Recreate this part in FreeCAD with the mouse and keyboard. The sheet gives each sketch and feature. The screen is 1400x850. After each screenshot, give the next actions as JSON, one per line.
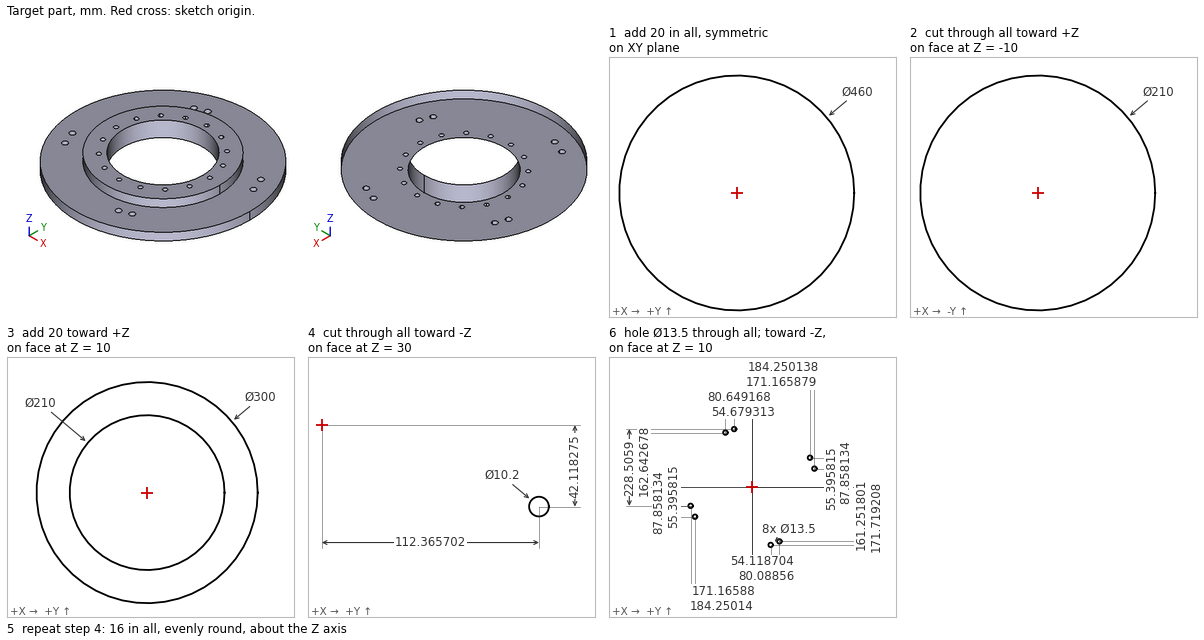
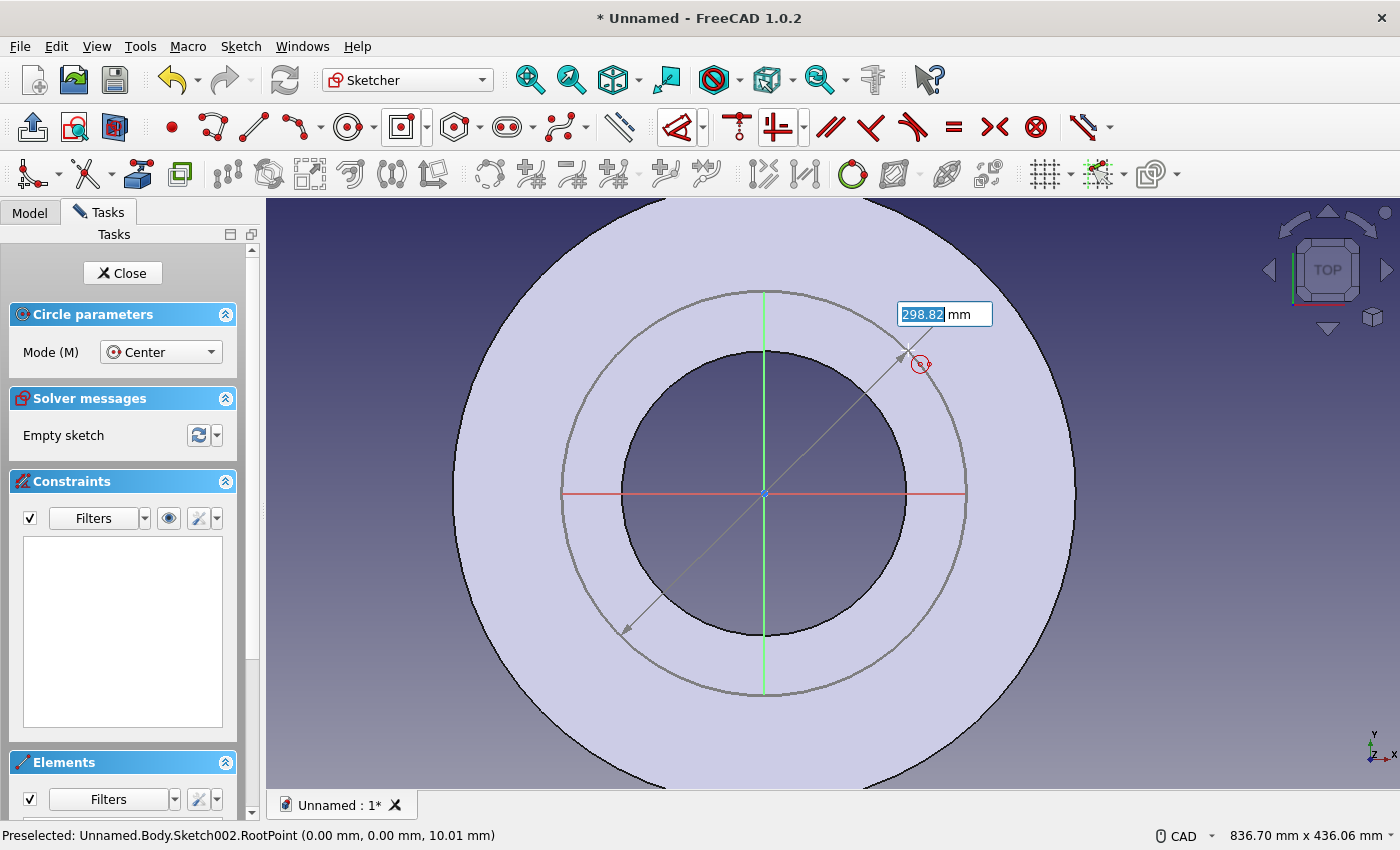
{"action": "type", "text": "300"}
{"action": "key", "text": "Return"}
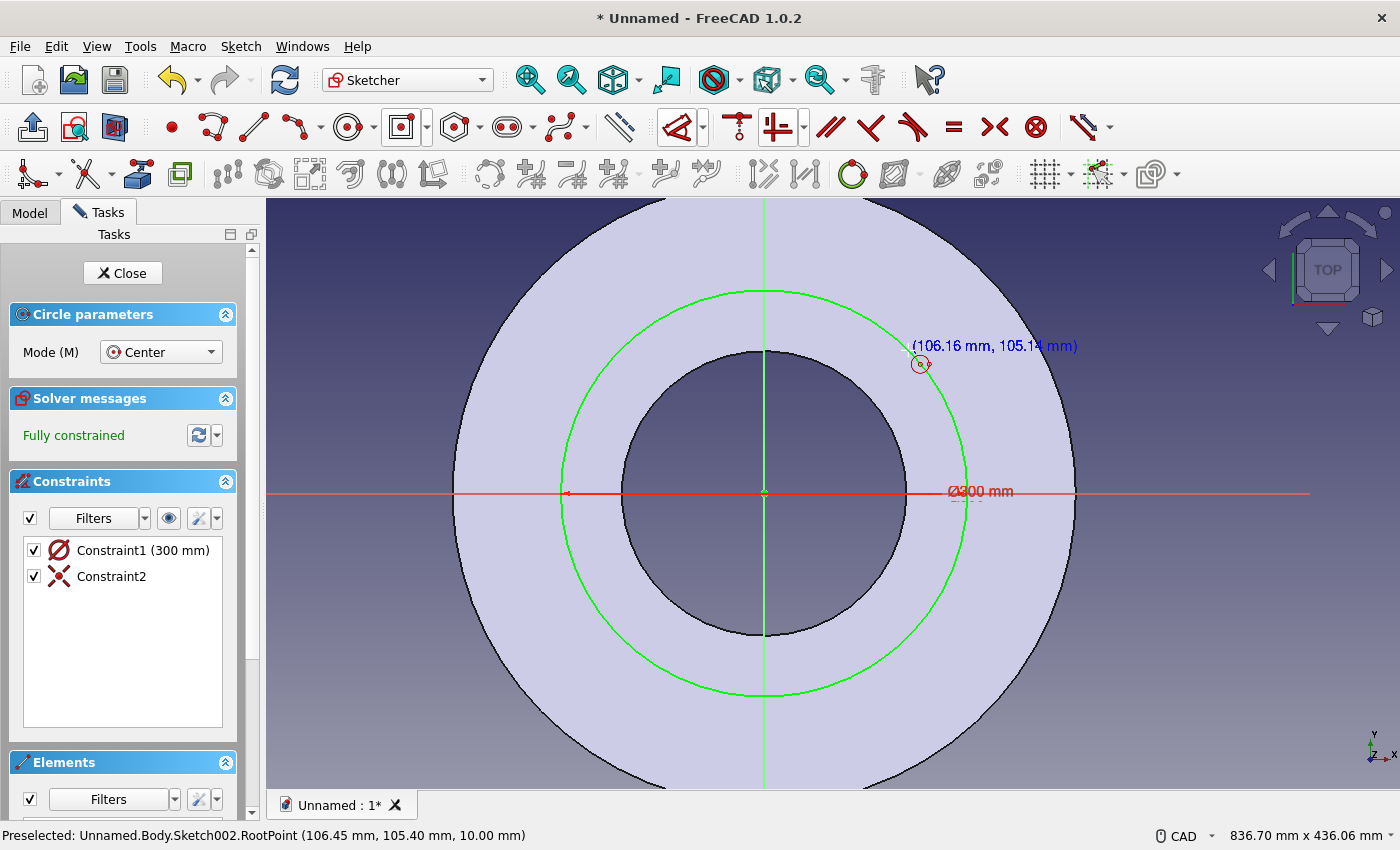
{"action": "left_click", "coordinate": [764, 493]}
{"action": "mouse_move", "coordinate": [865, 393]}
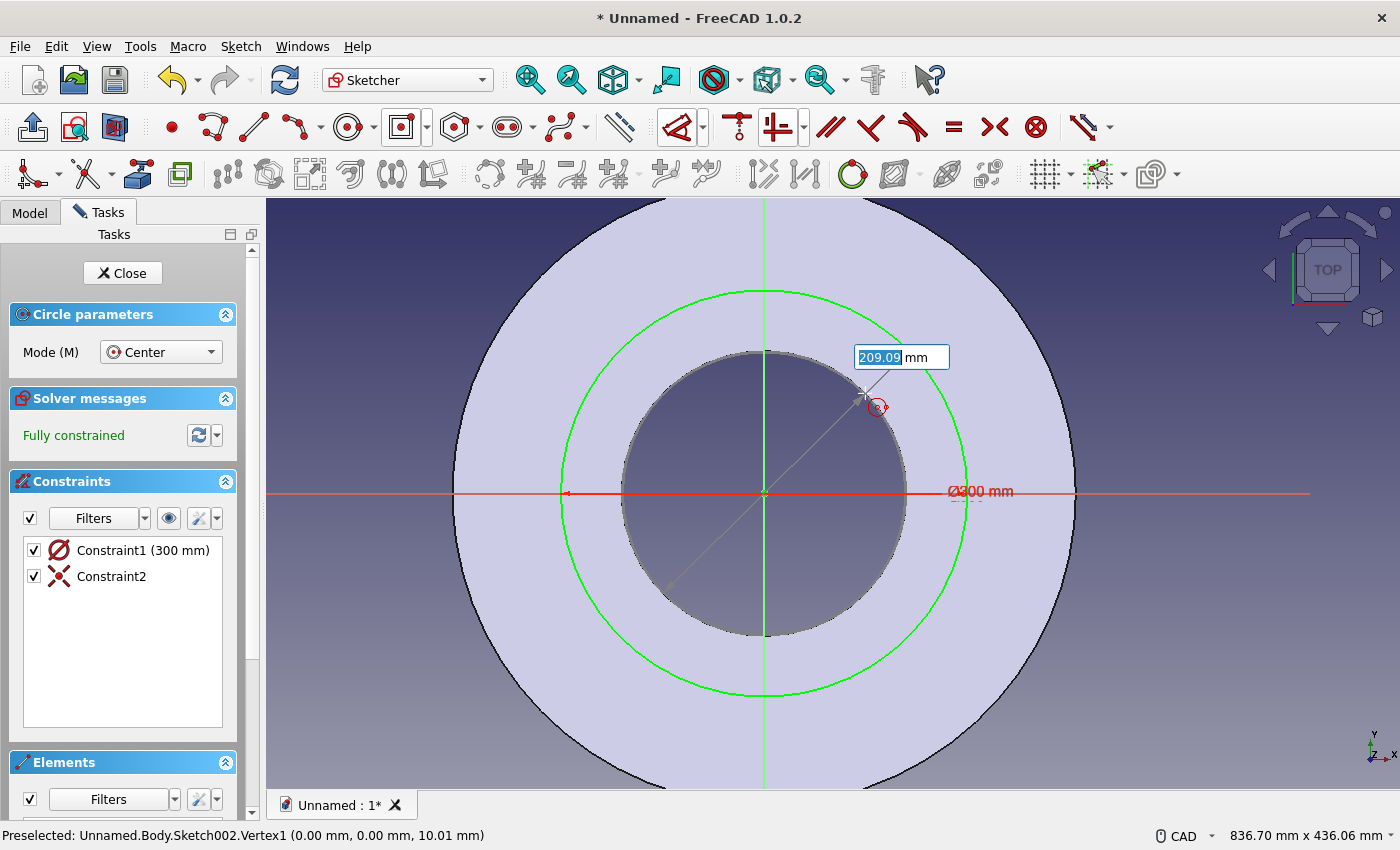
{"action": "type", "text": "210"}
{"action": "key", "text": "Return"}
{"action": "key", "text": "Escape"}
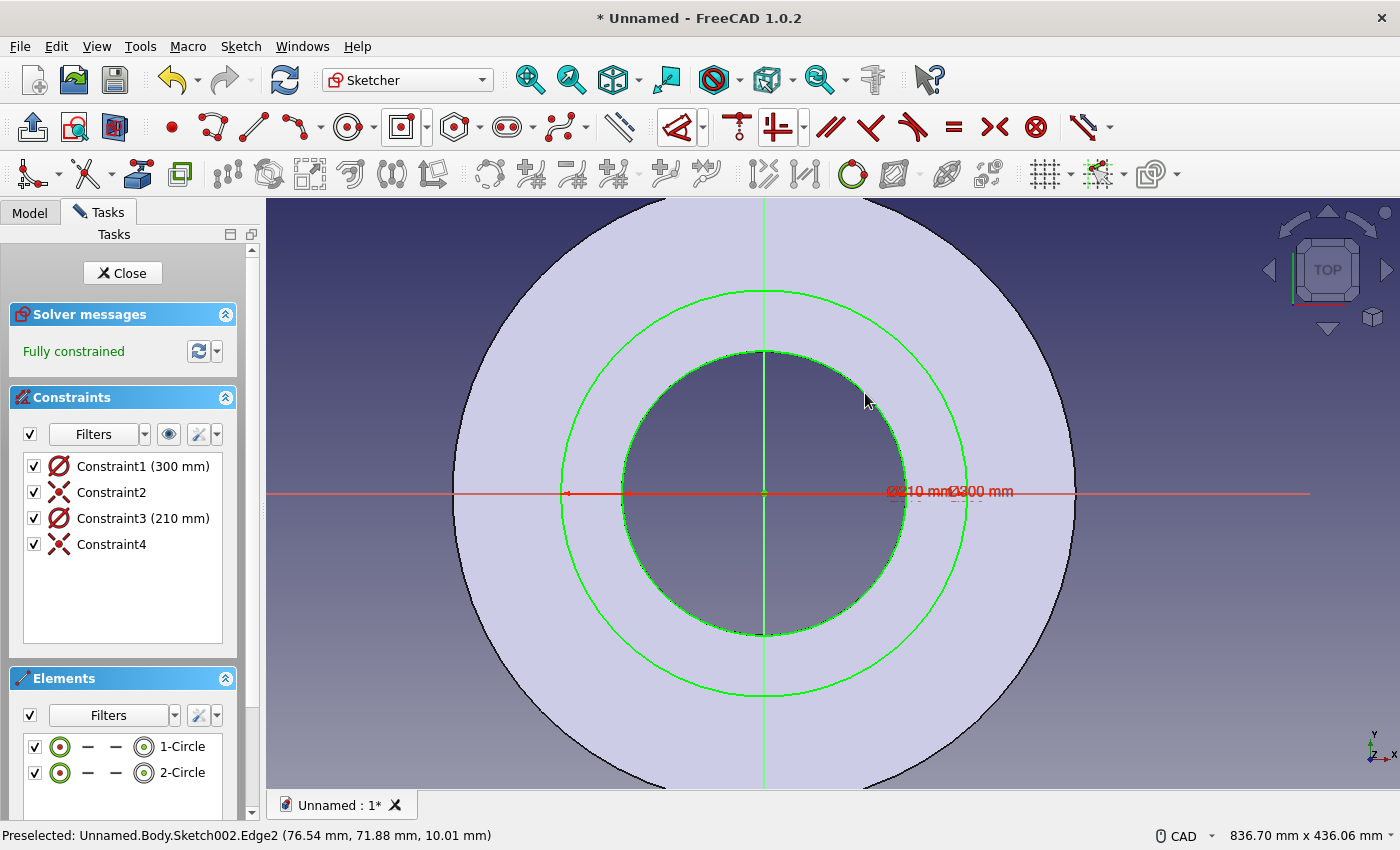
{"action": "left_click", "coordinate": [123, 273]}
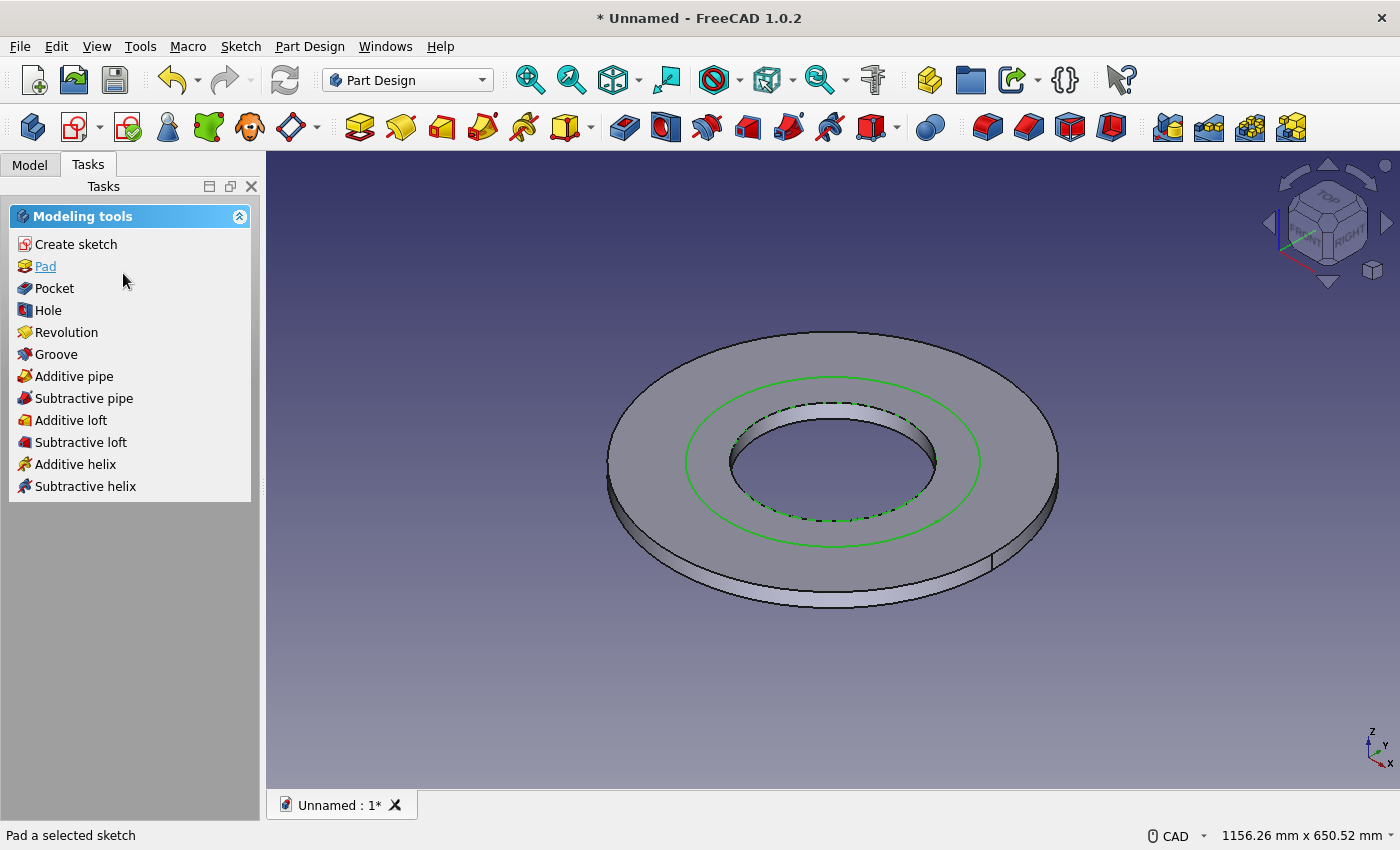
{"action": "left_click", "coordinate": [360, 128]}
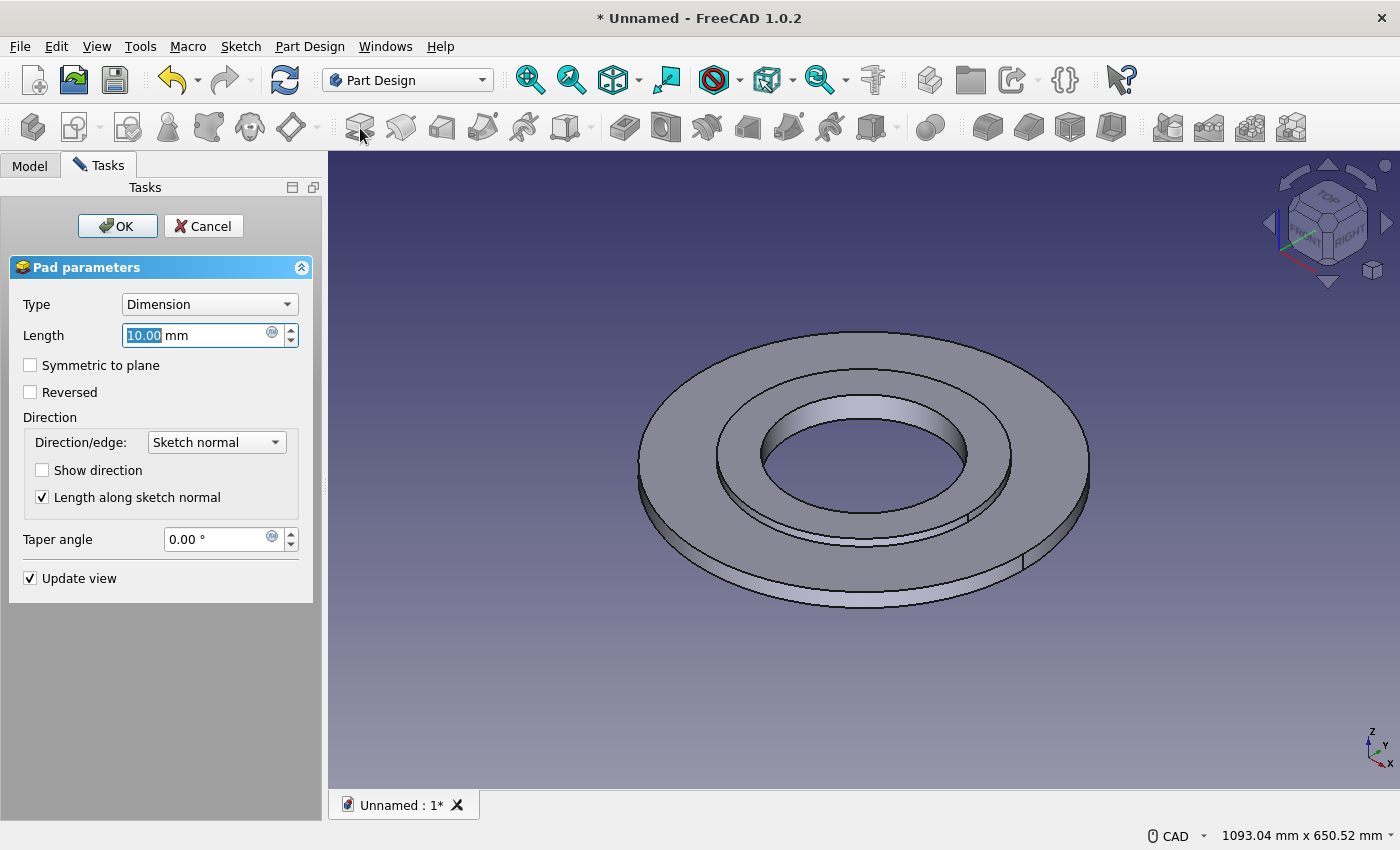
{"action": "type", "text": "20"}
{"action": "key", "text": "Tab"}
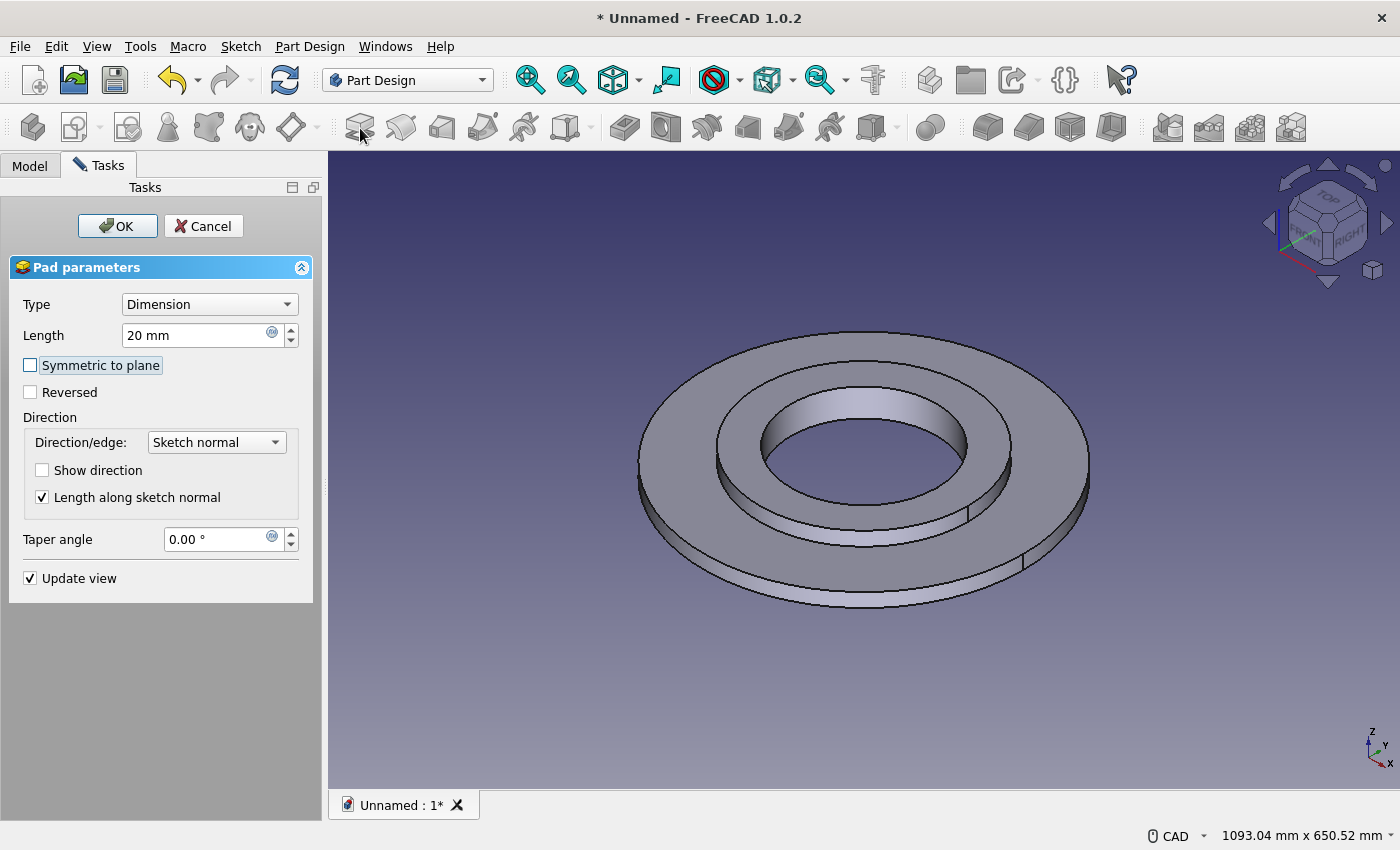
{"action": "left_click", "coordinate": [118, 226]}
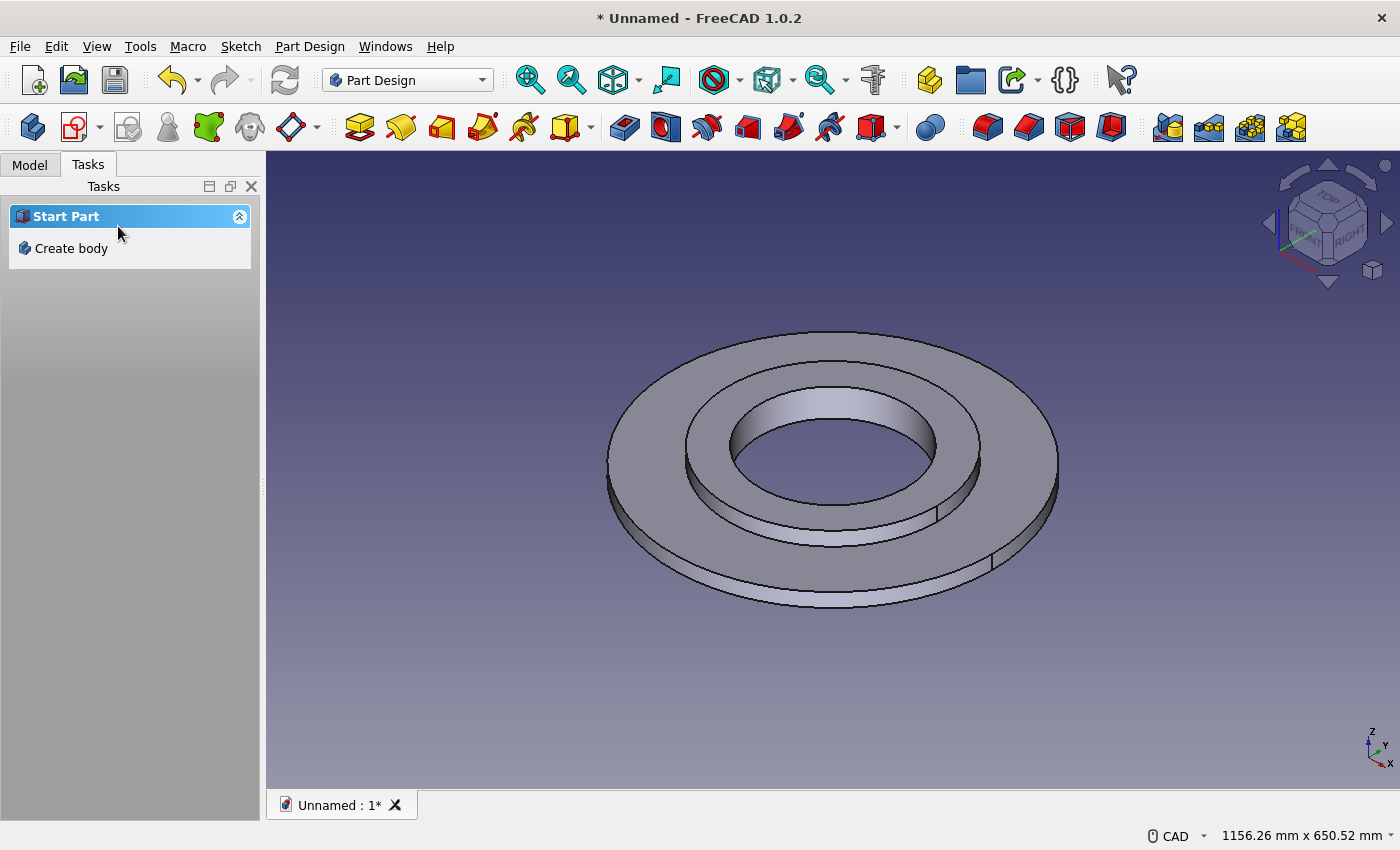
{"action": "left_click", "coordinate": [922, 496]}